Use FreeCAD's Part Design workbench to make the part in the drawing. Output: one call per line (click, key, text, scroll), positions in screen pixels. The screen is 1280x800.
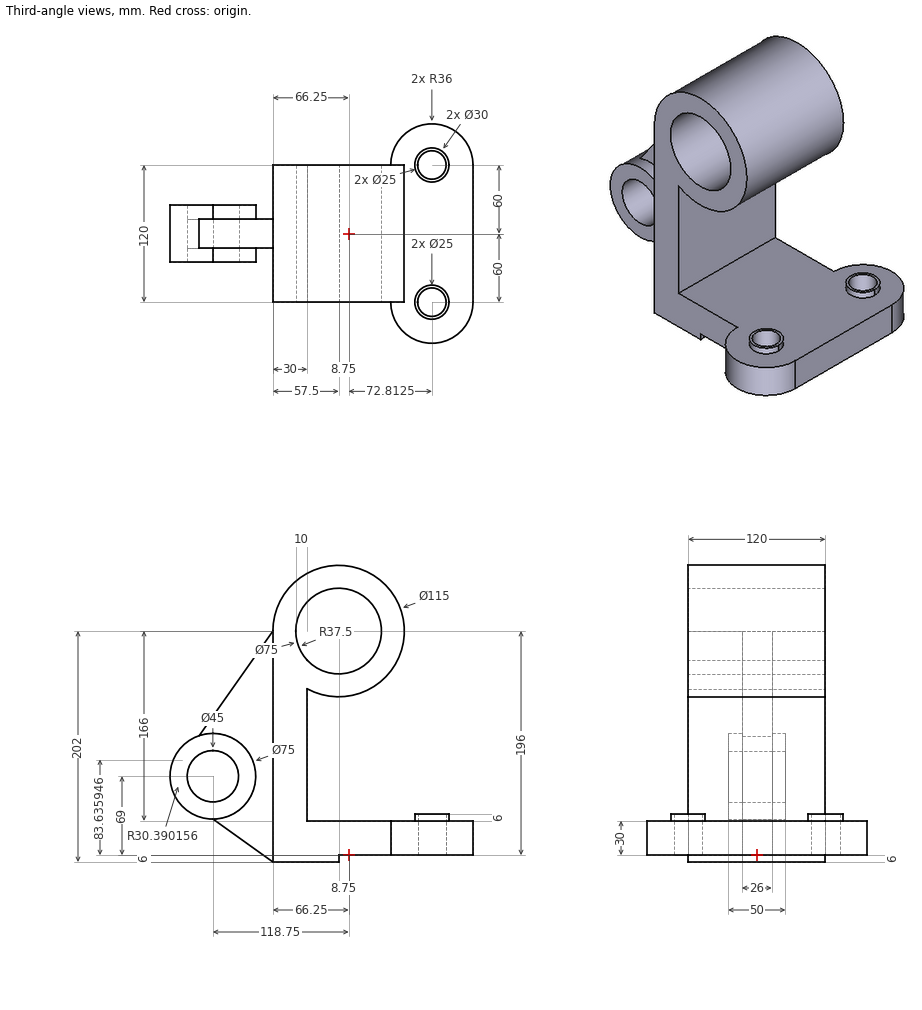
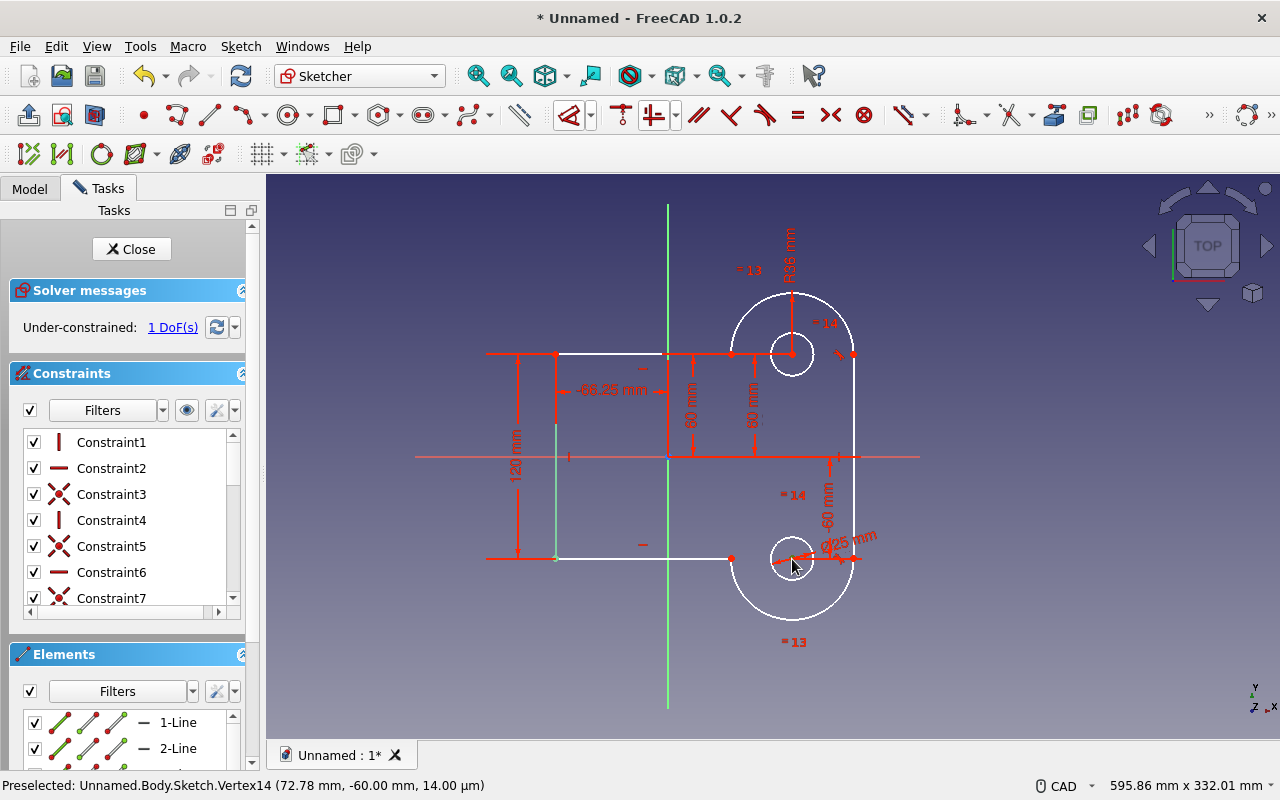
key(l)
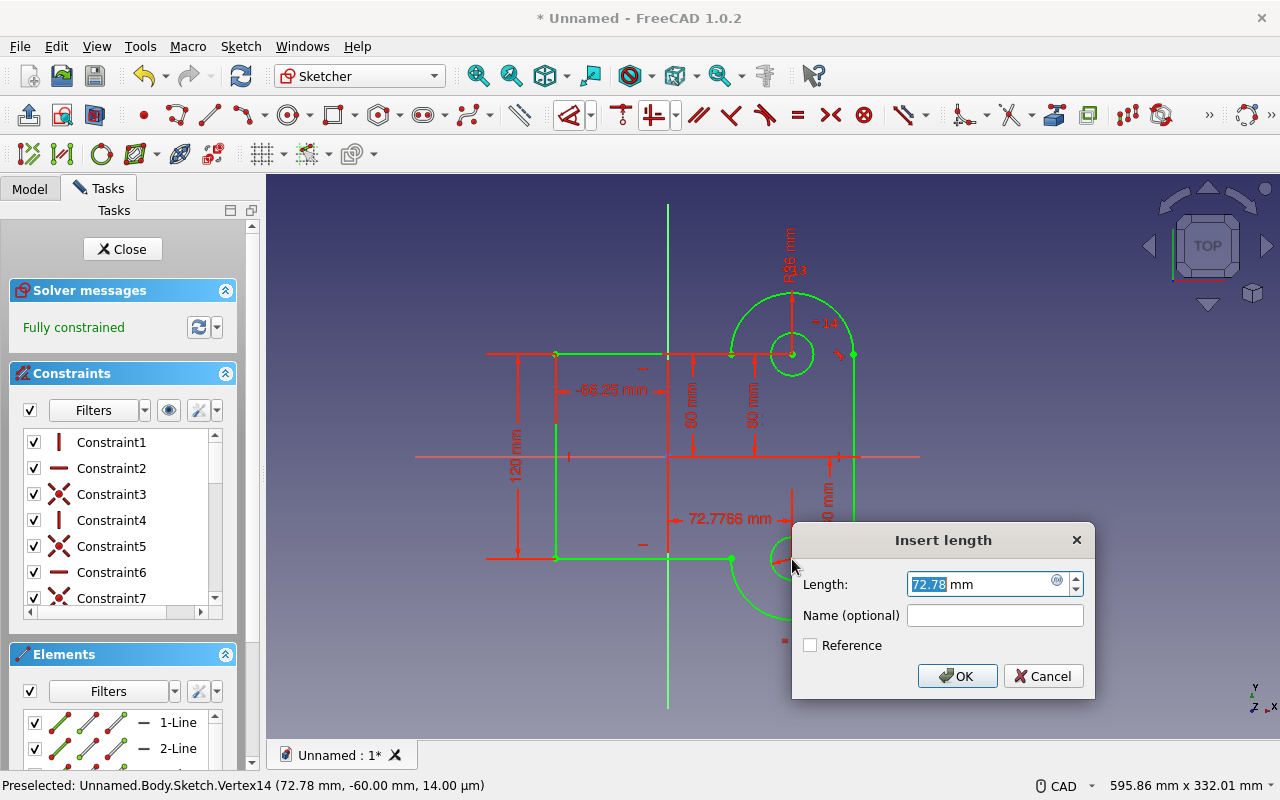
text(72.8125)
key(Return)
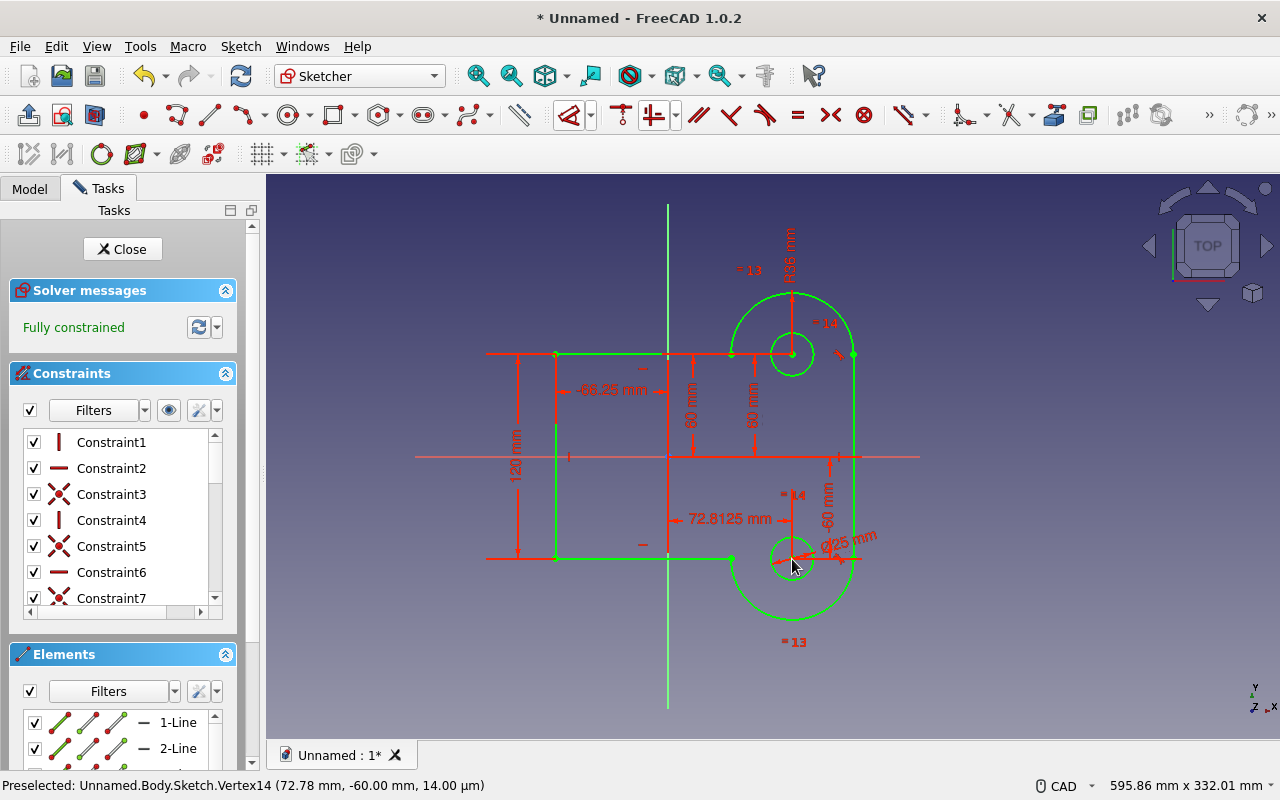
click(123, 249)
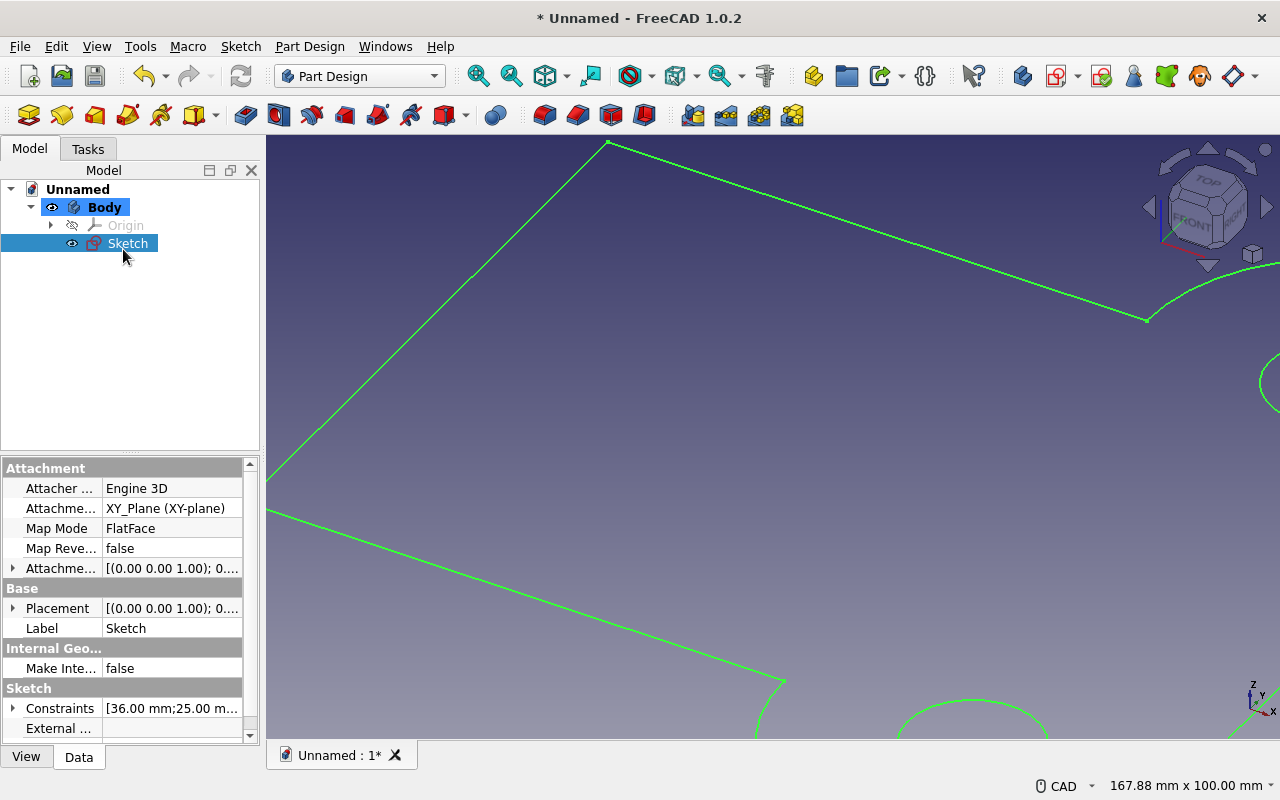
click(29, 116)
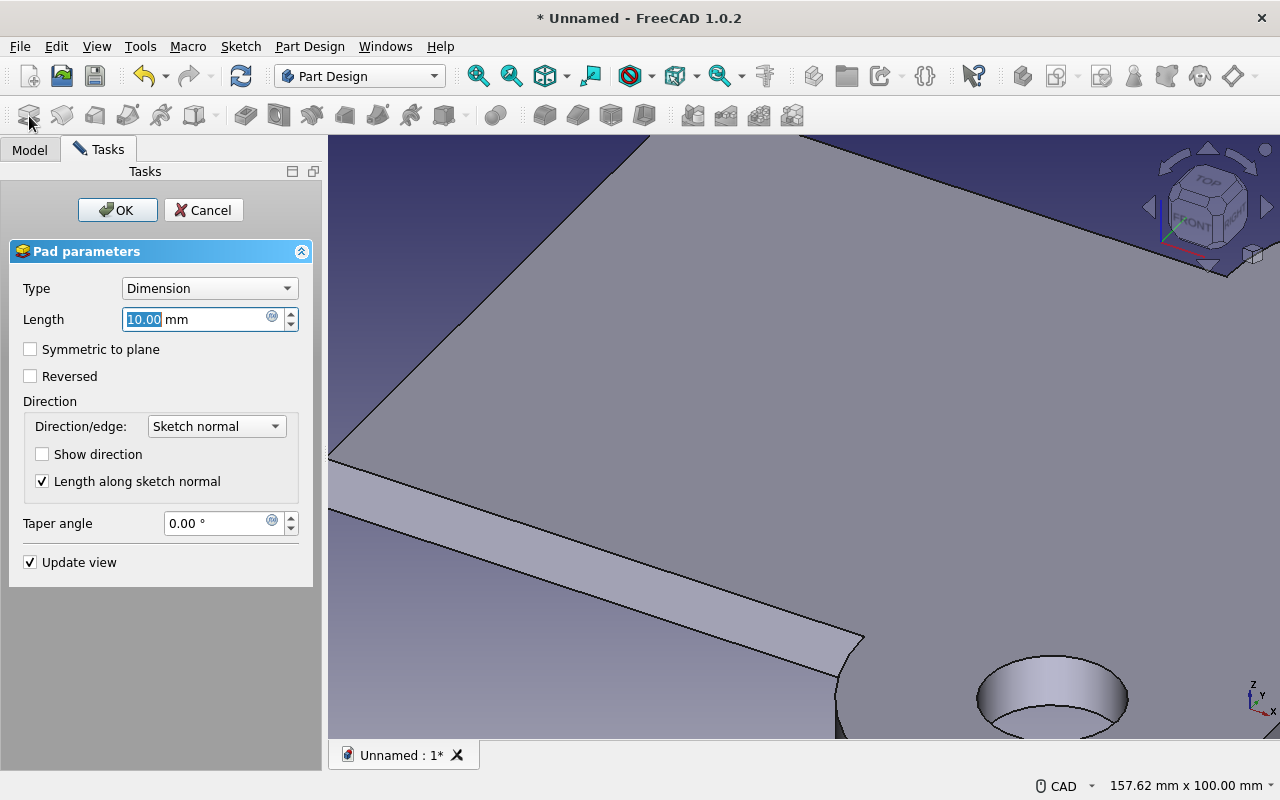
text(30)
key(Tab)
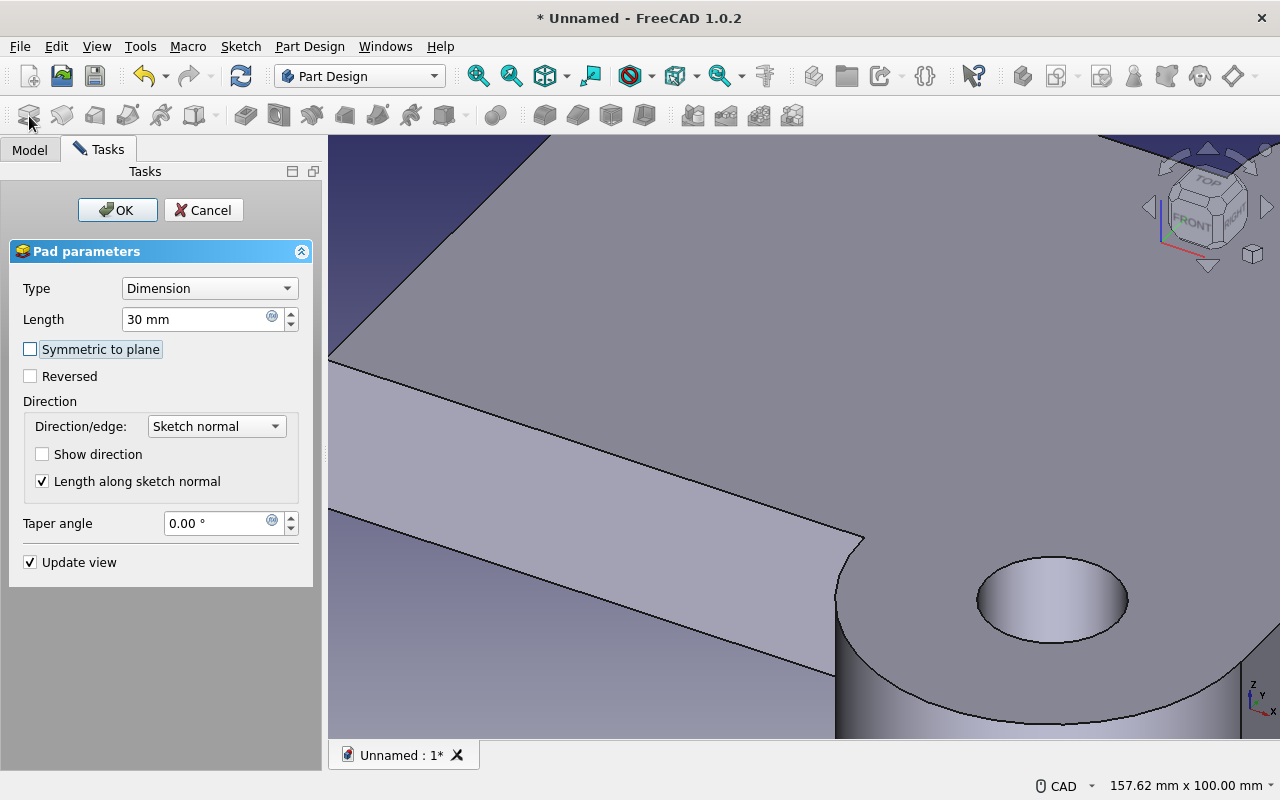
click(118, 210)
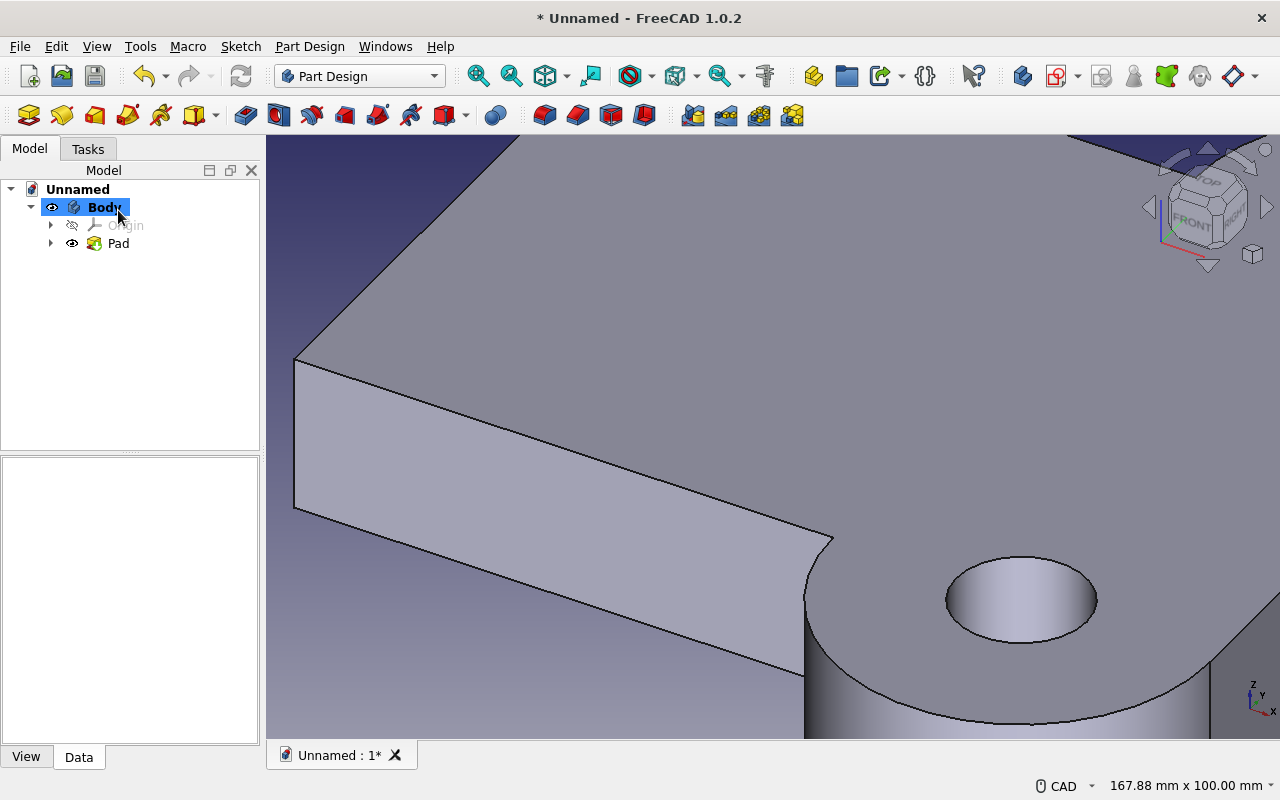
key(v)
key(f)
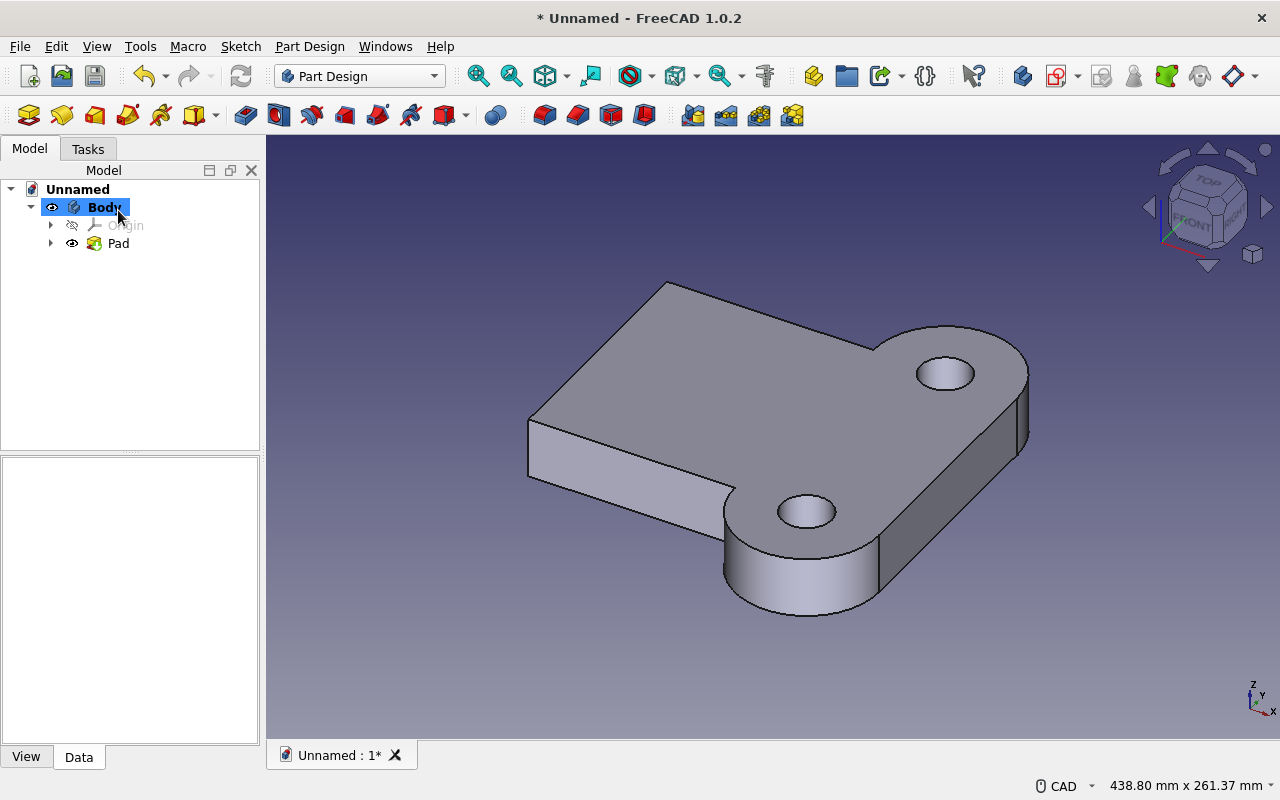
click(773, 408)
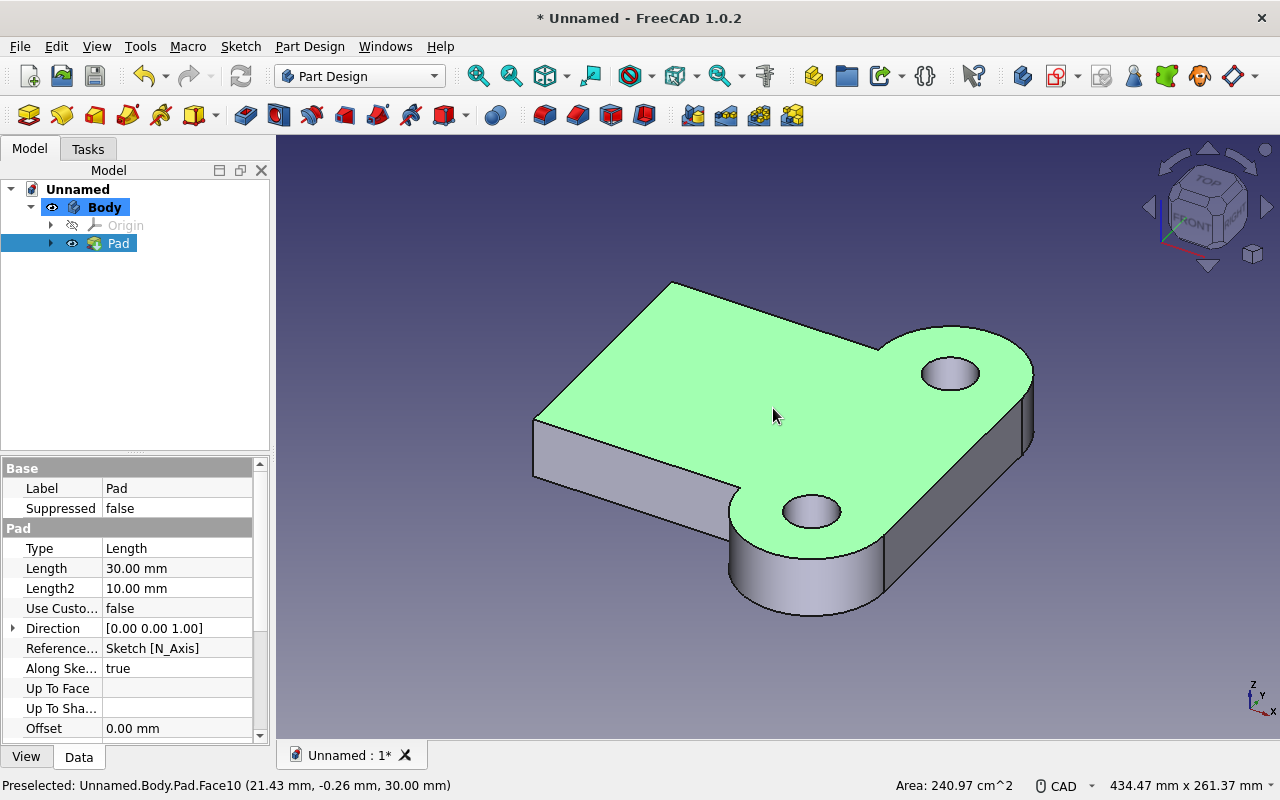
click(1056, 76)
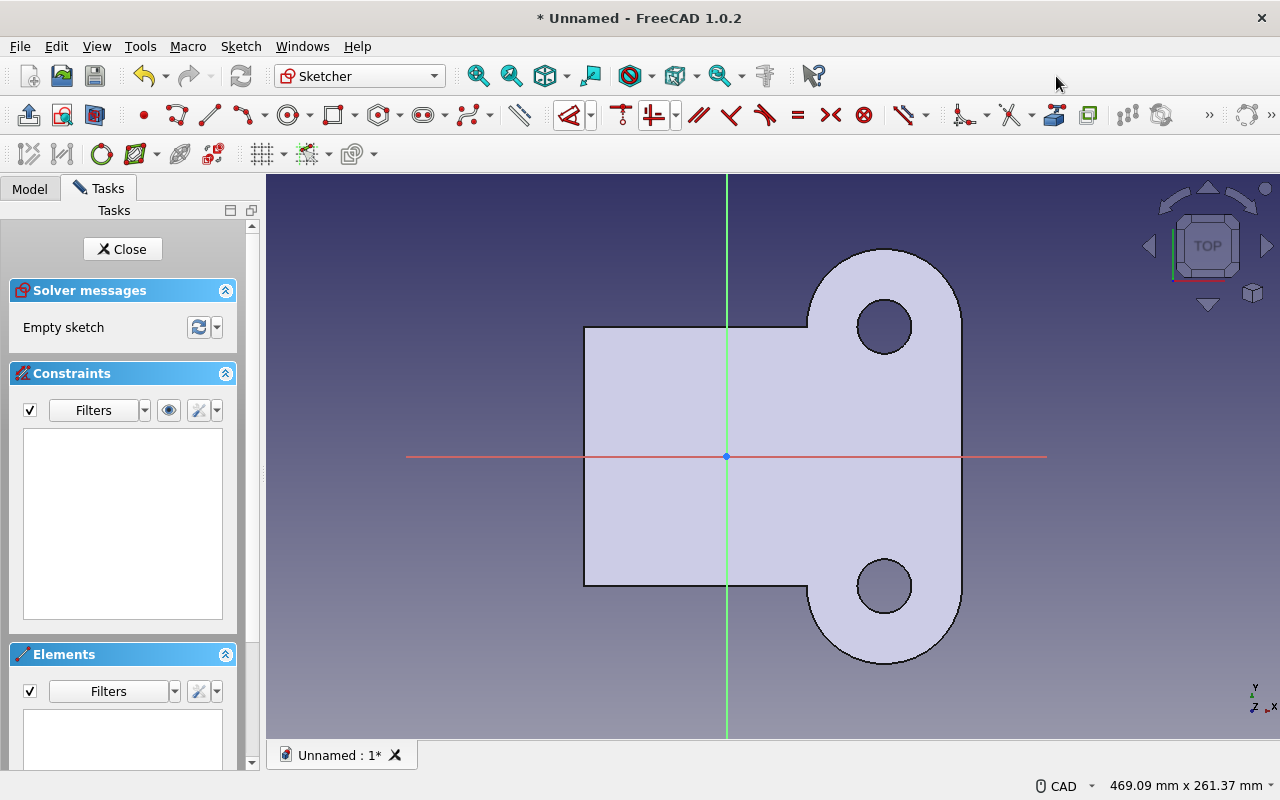
key(g)
key(c)